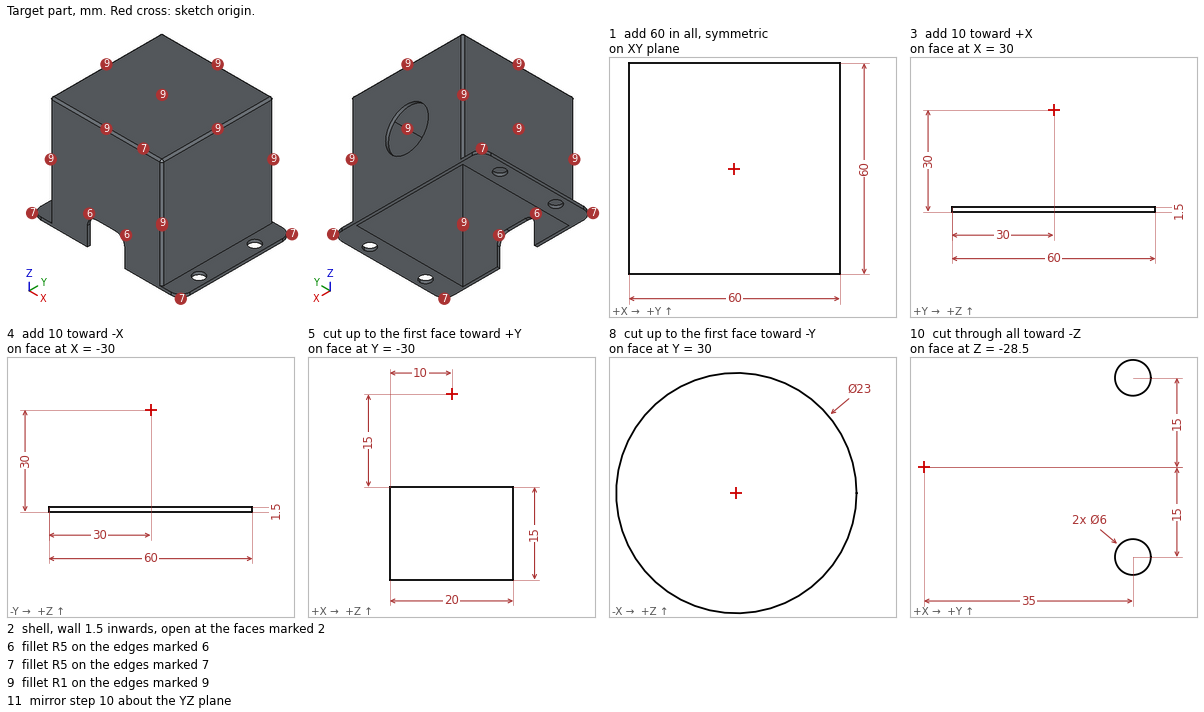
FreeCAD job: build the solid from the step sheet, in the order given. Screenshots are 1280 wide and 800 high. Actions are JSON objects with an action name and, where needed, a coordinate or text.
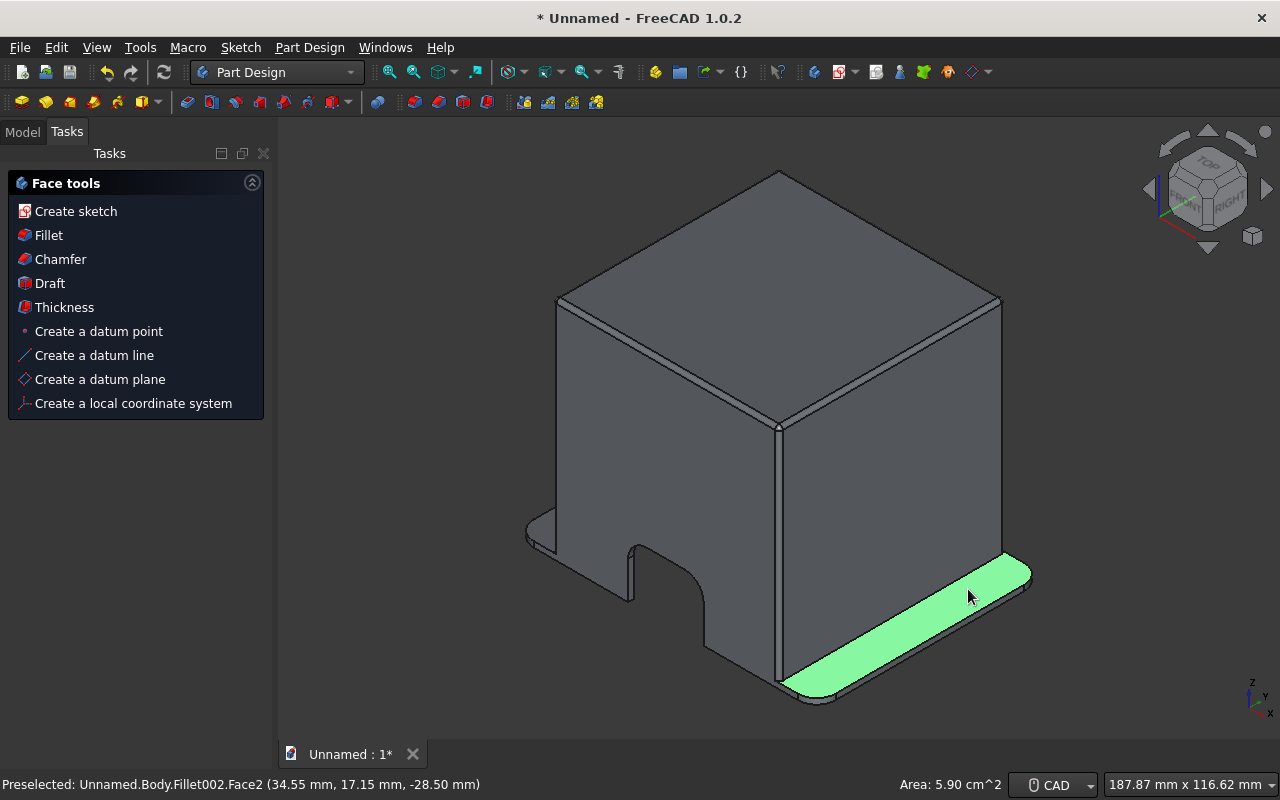
{"action": "left_click", "coordinate": [840, 72]}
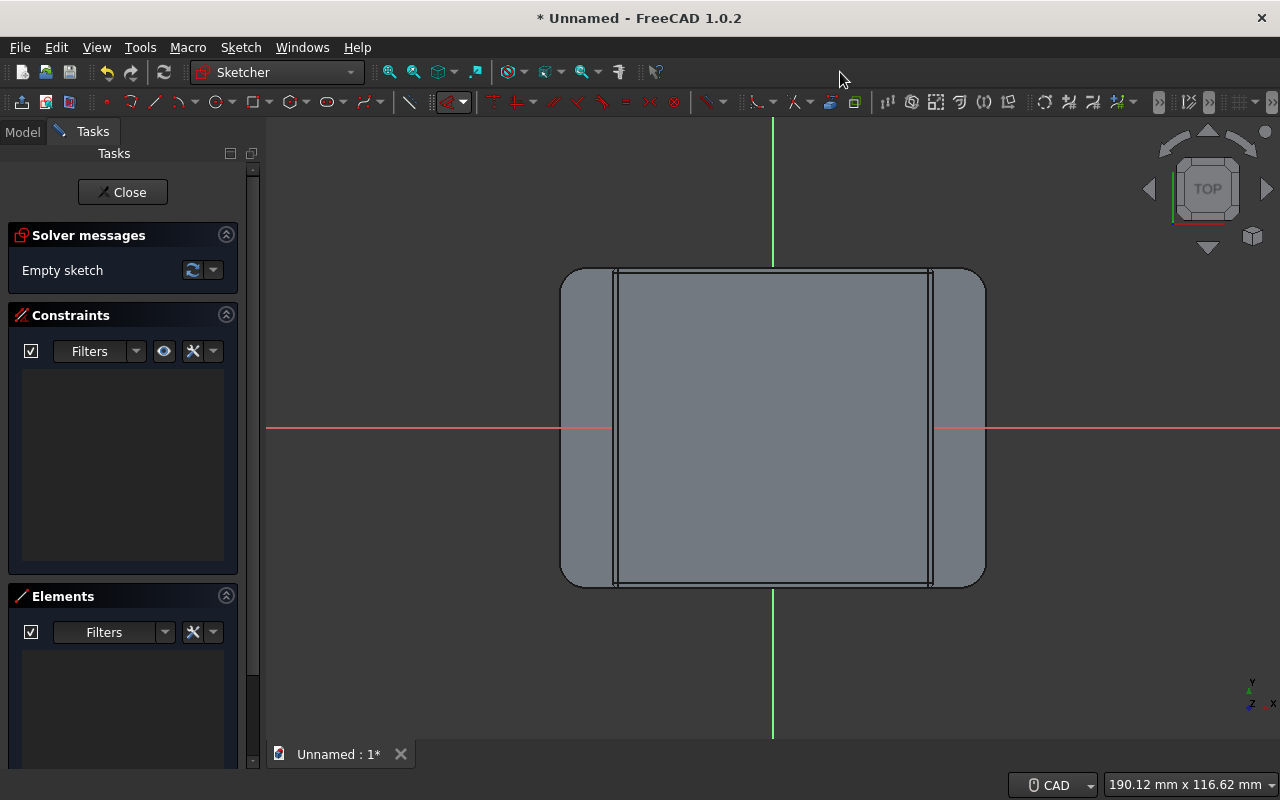
{"action": "key", "text": "q s"}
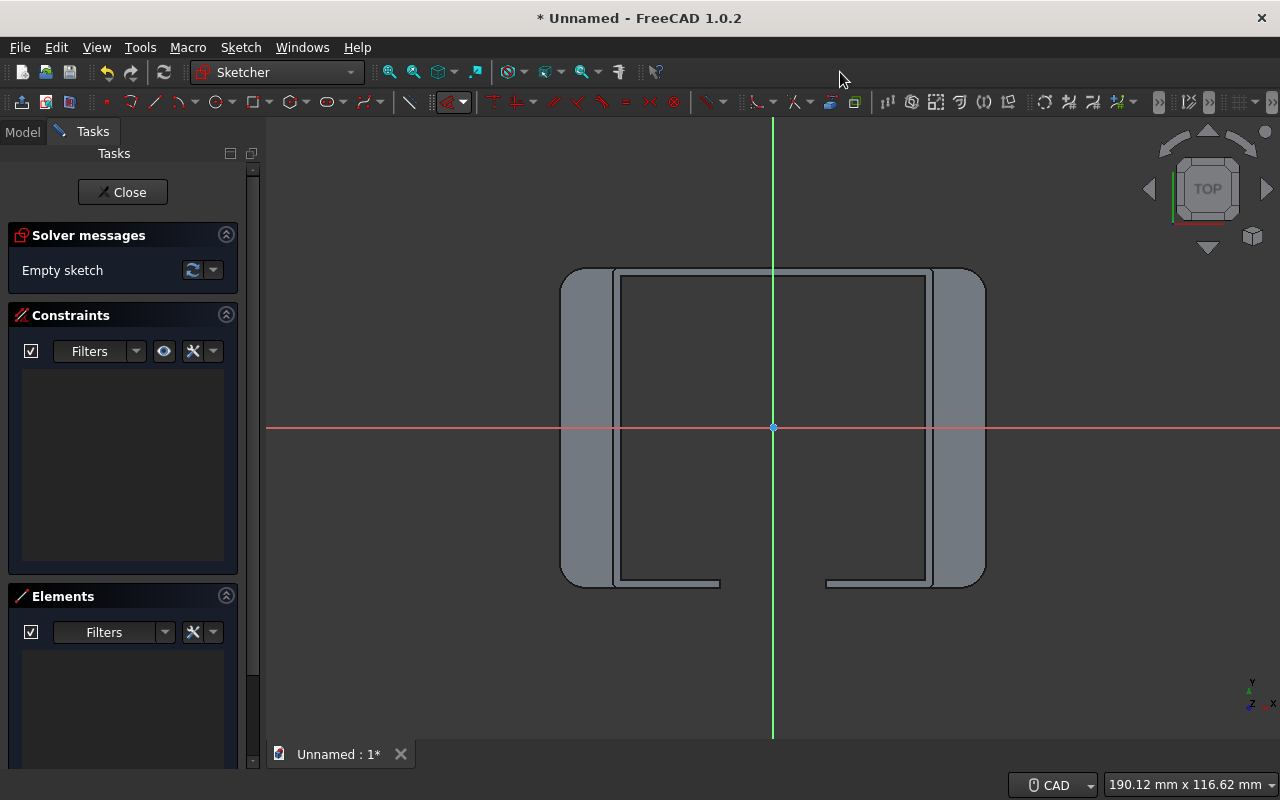
{"action": "scroll", "coordinate": [1013, 428], "scroll_direction": "up", "scroll_amount": 4}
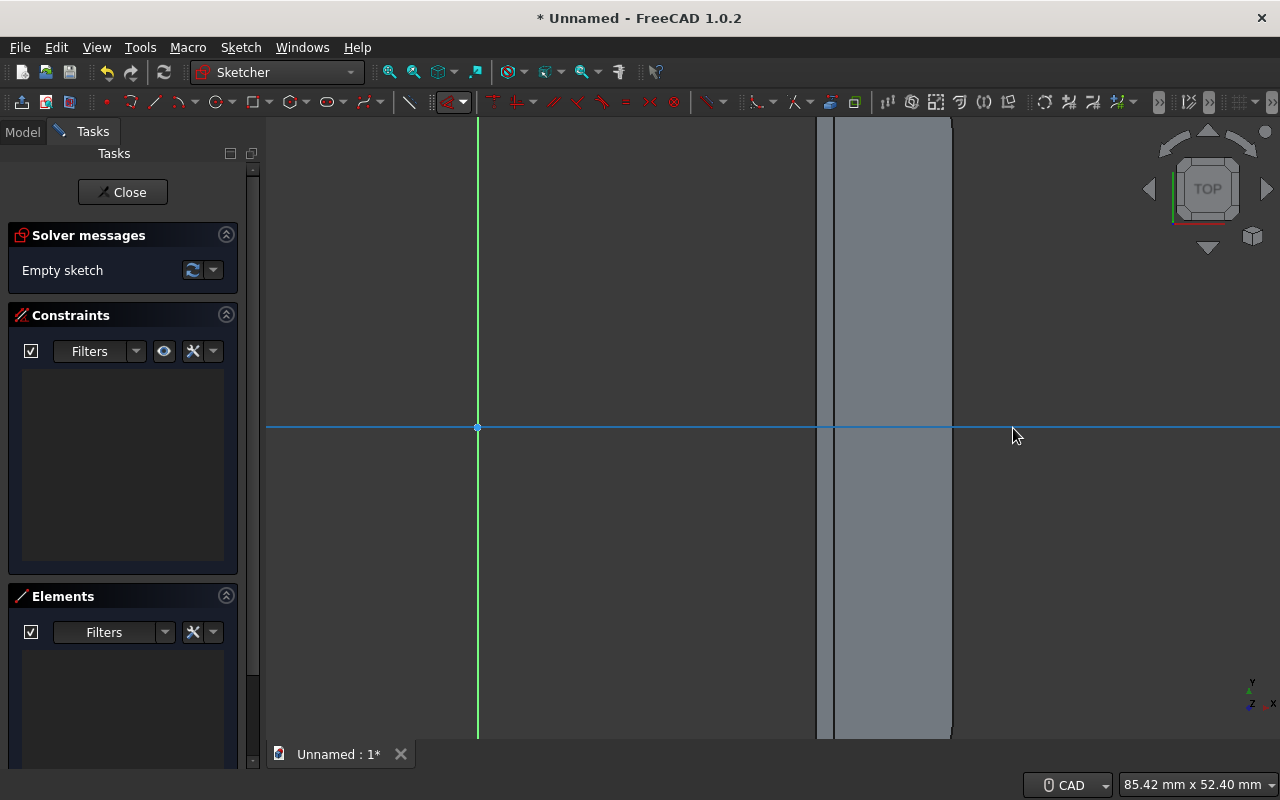
{"action": "left_click", "coordinate": [216, 102]}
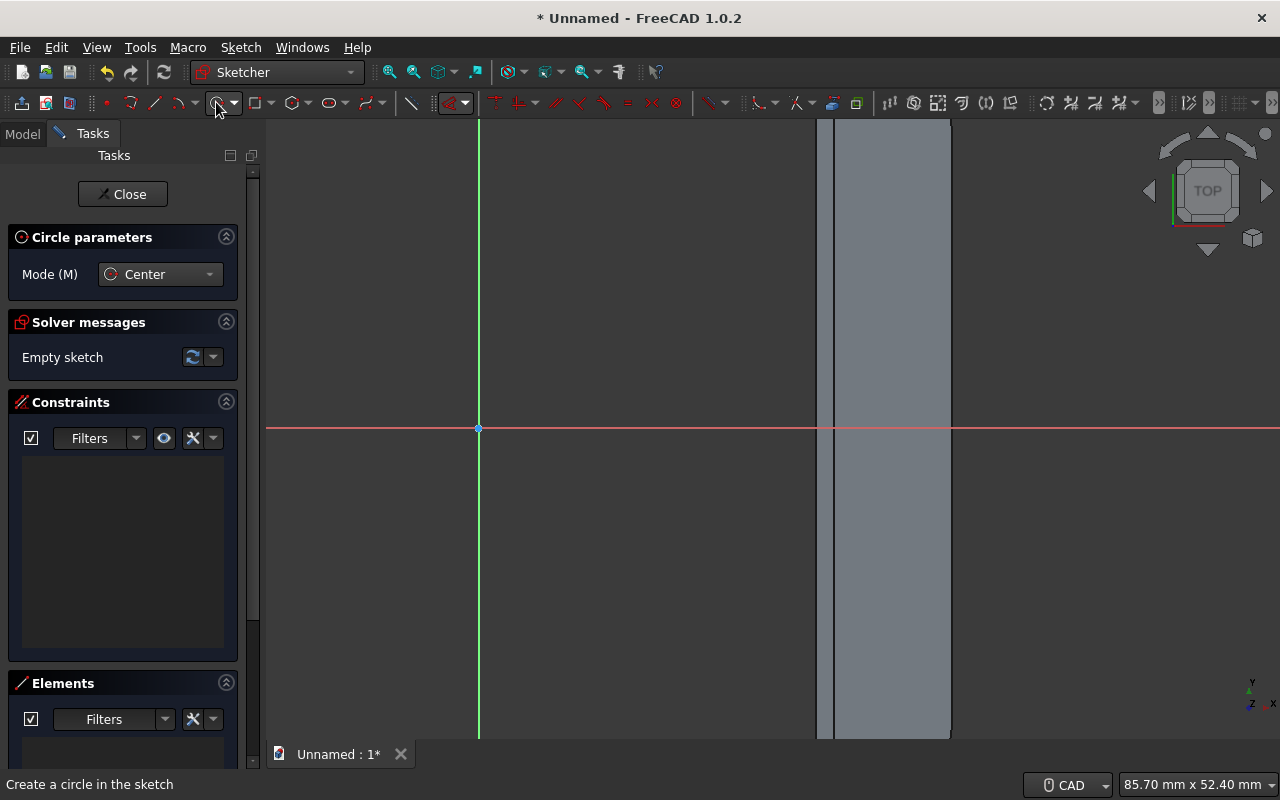
{"action": "left_click", "coordinate": [893, 606]}
{"action": "mouse_move", "coordinate": [918, 581]}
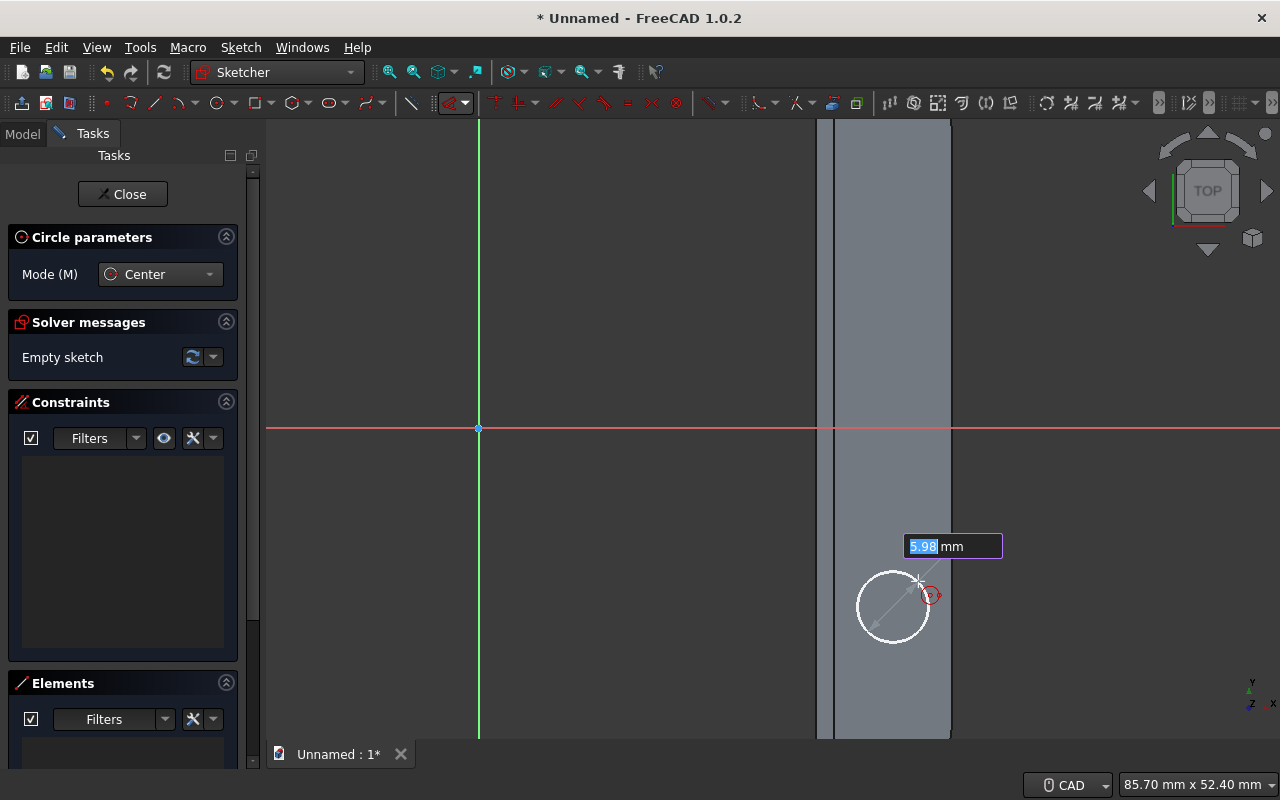
{"action": "type", "text": "6"}
{"action": "key", "text": "Return"}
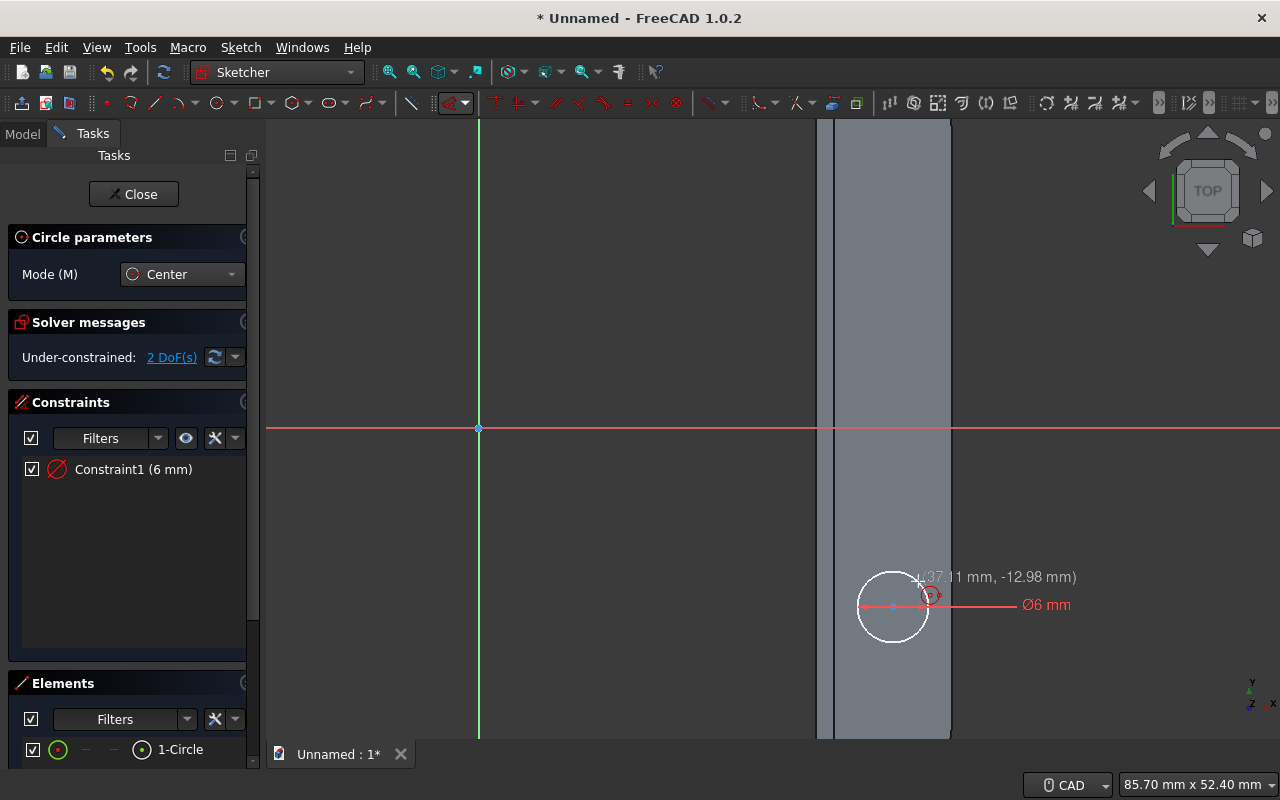
{"action": "left_click", "coordinate": [893, 251]}
{"action": "mouse_move", "coordinate": [918, 226]}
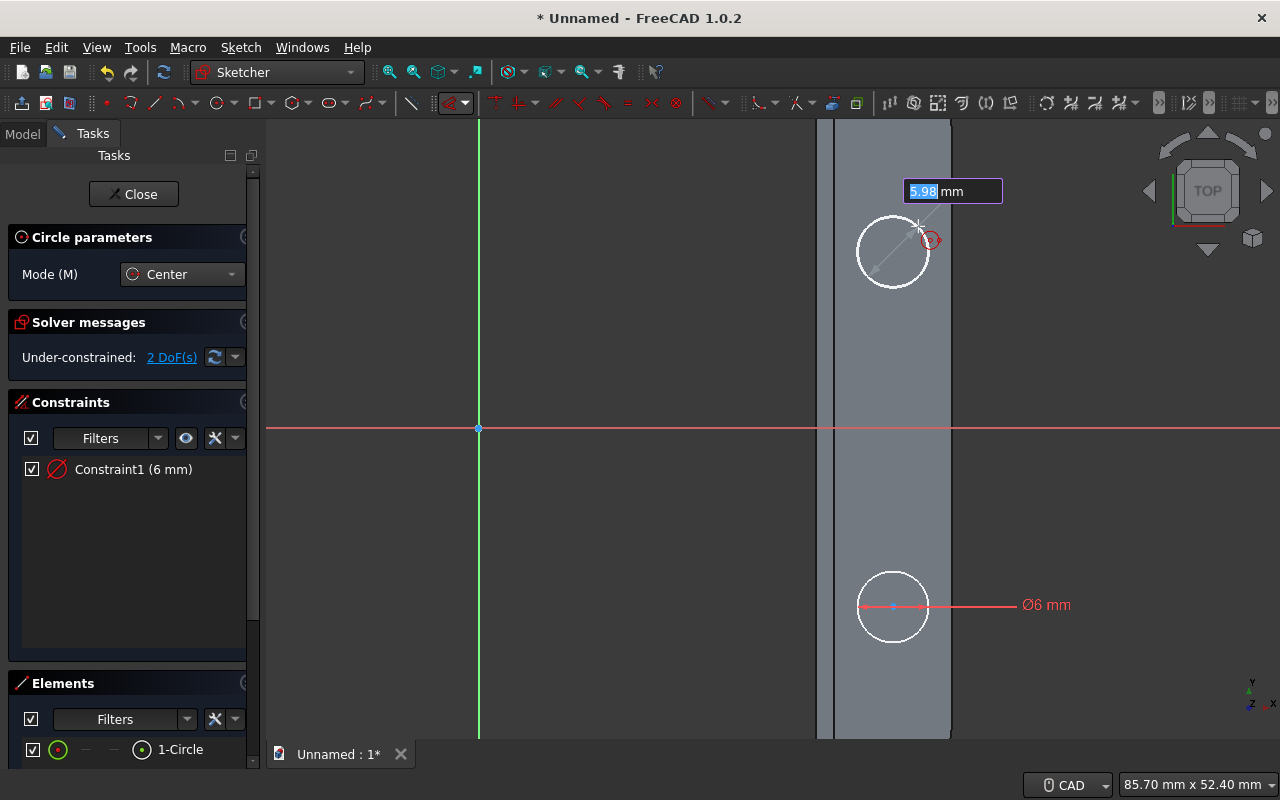
{"action": "type", "text": "6"}
{"action": "key", "text": "Return"}
{"action": "key", "text": "Escape"}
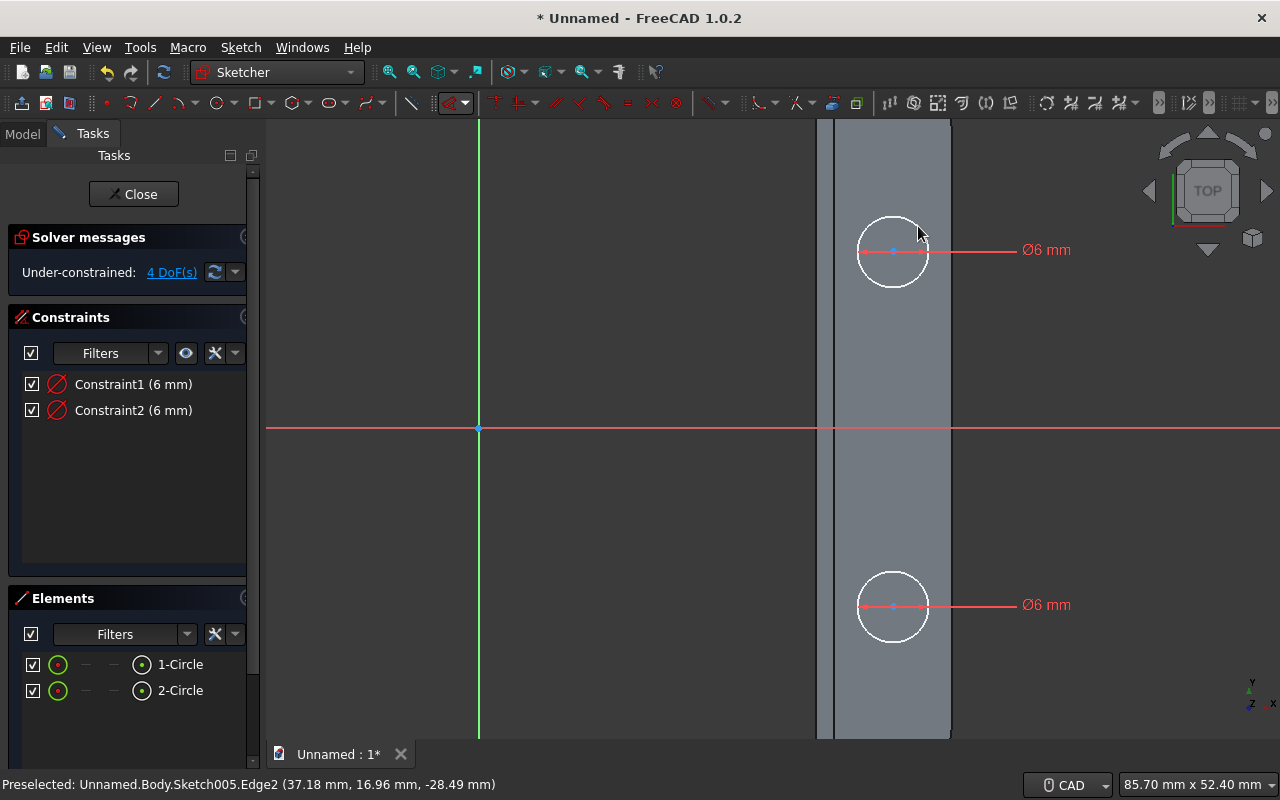
{"action": "left_click", "coordinate": [893, 607]}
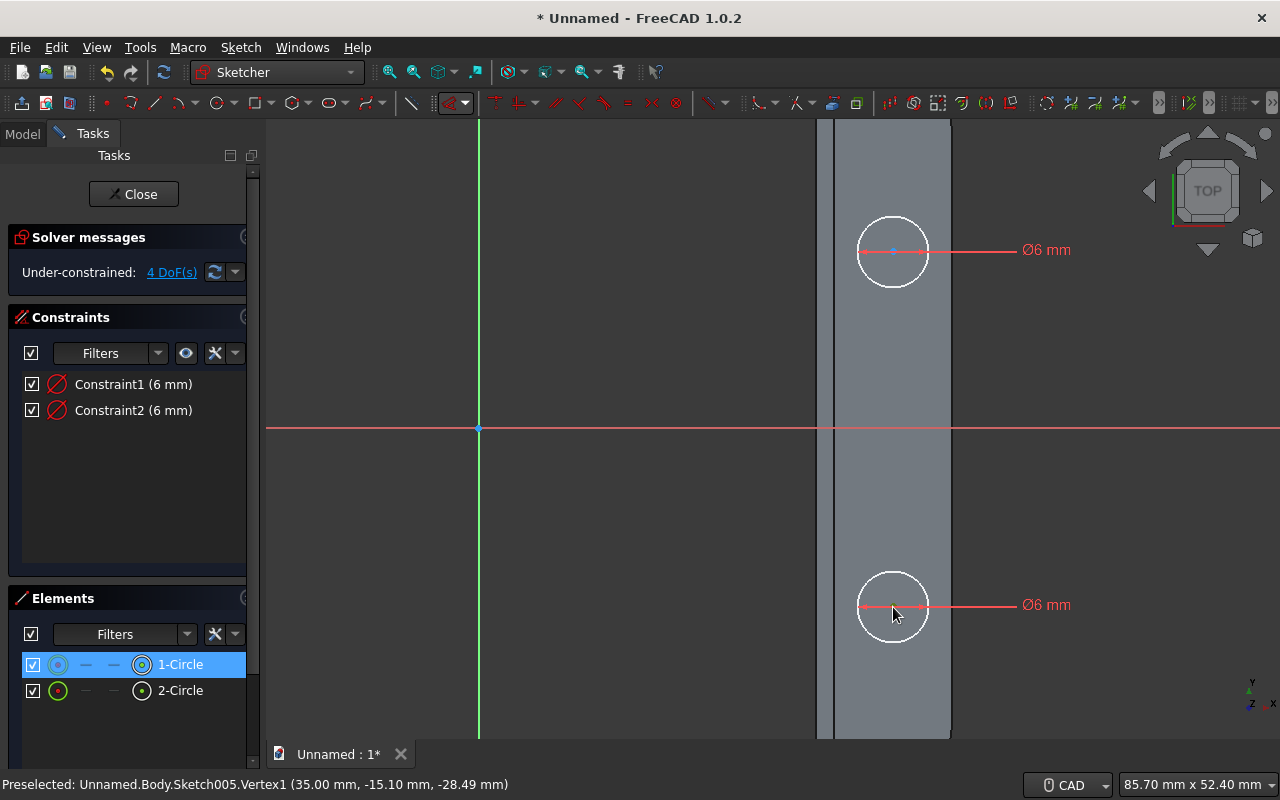
{"action": "left_click", "coordinate": [893, 252]}